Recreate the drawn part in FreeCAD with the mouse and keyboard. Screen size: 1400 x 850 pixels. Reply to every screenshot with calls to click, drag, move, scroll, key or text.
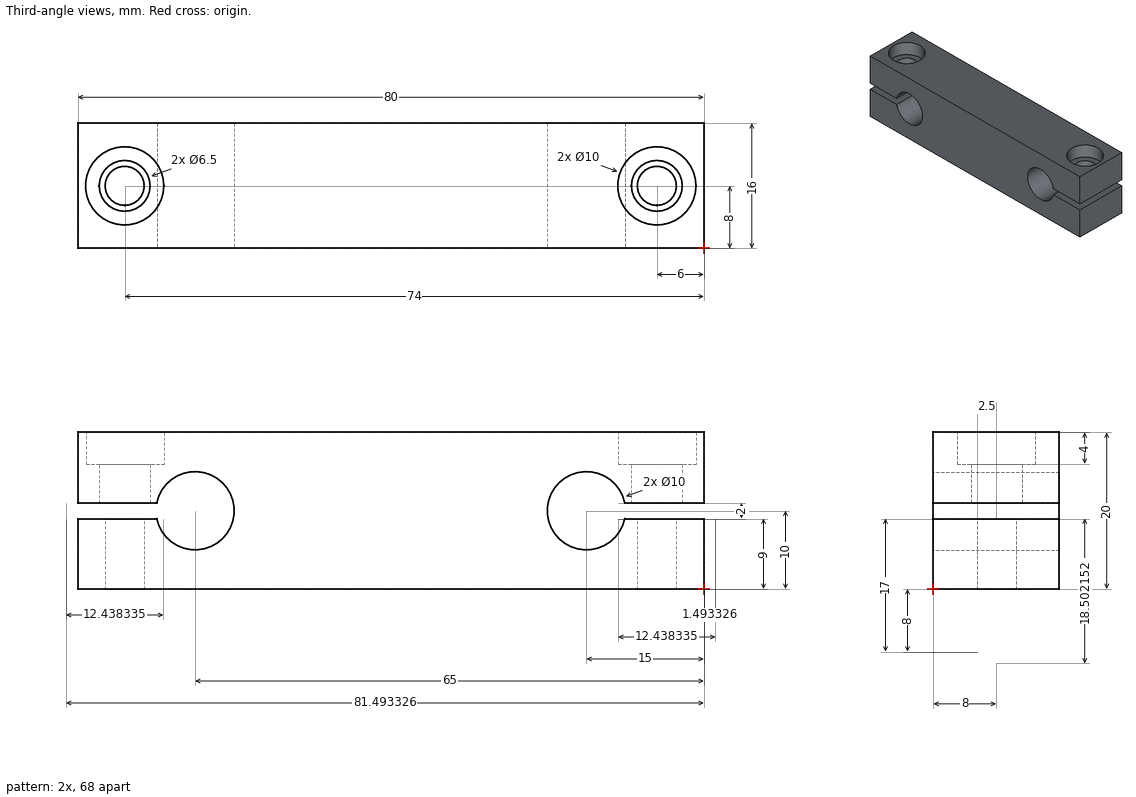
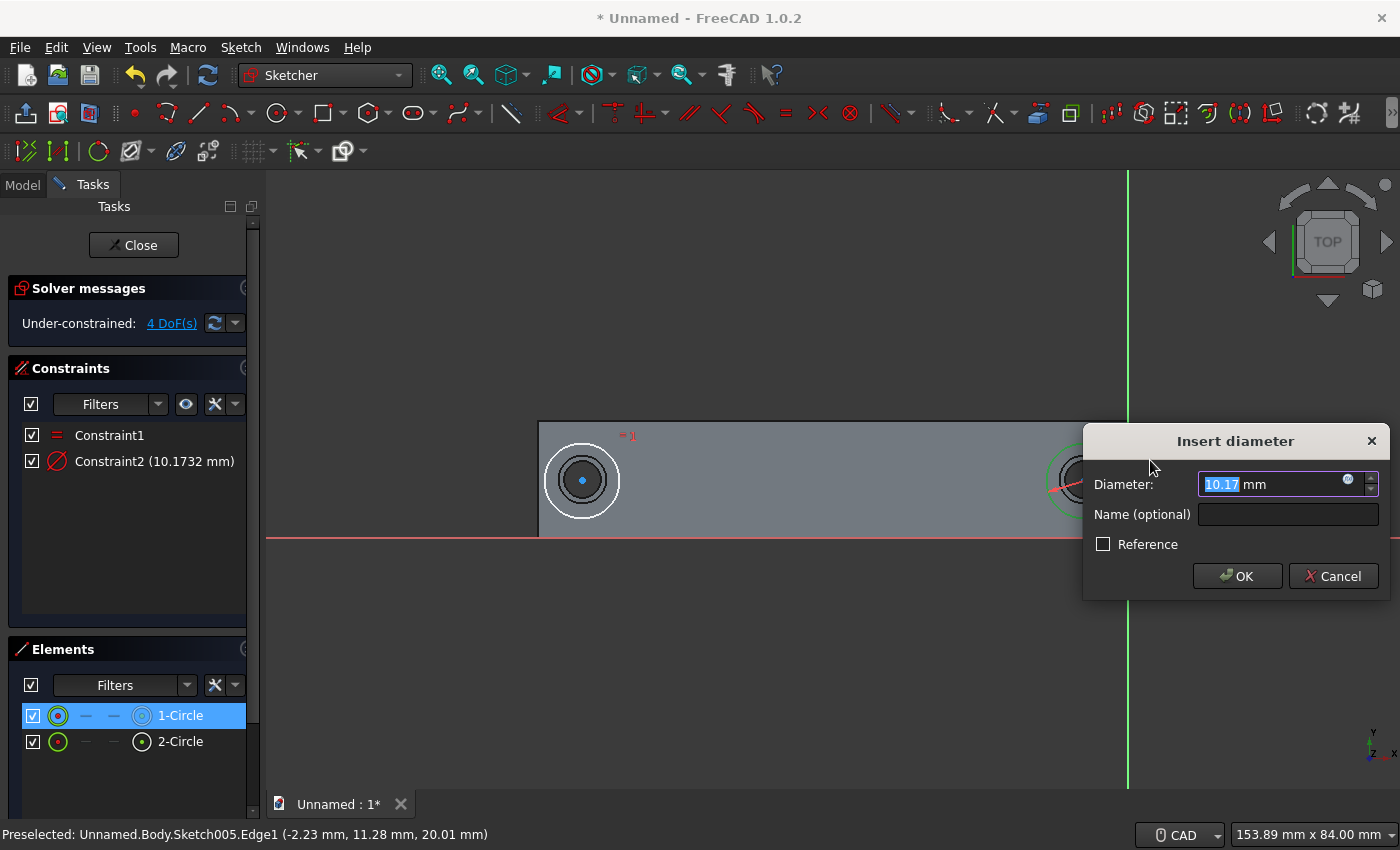
text(10)
key(Return)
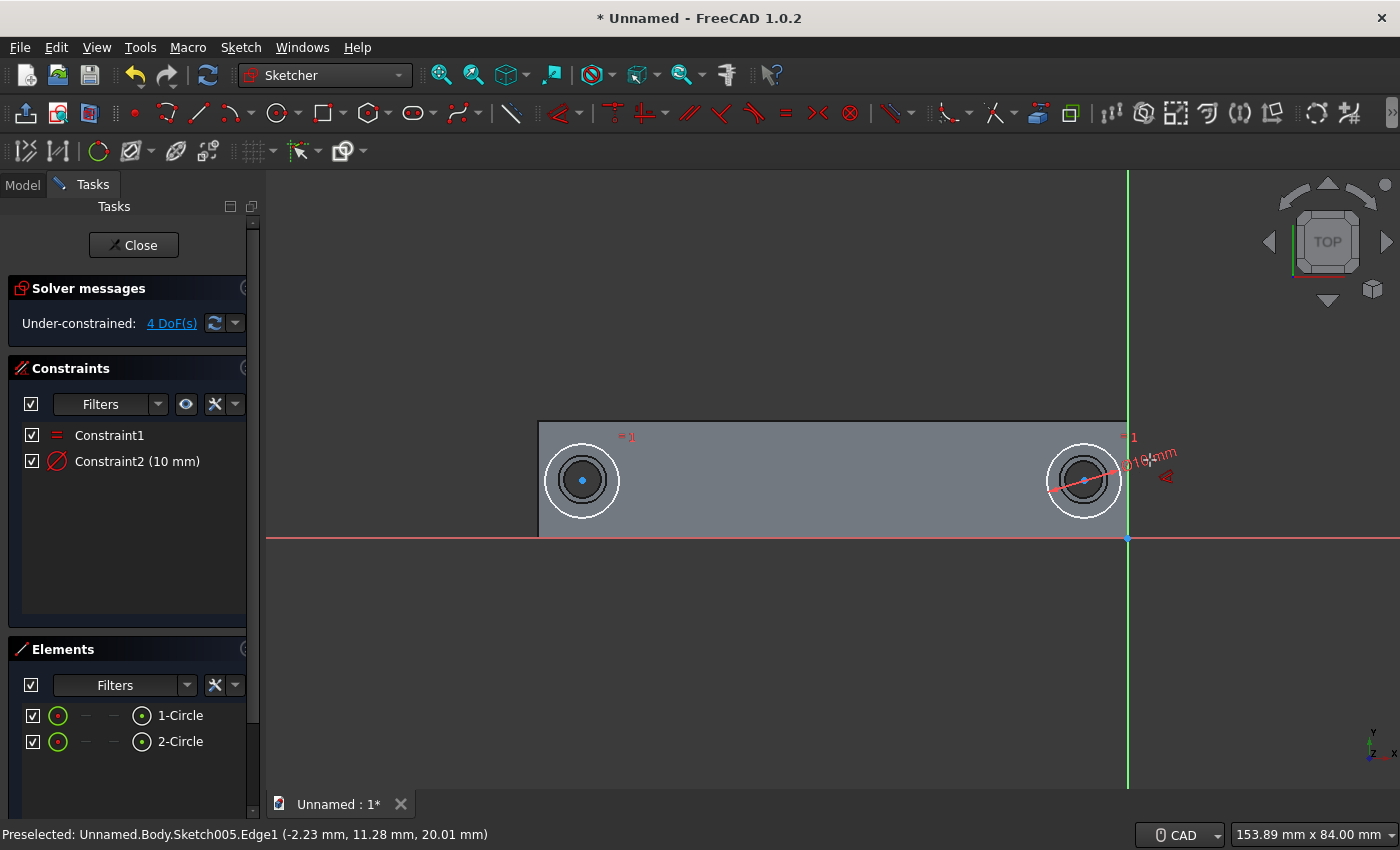
click(1084, 481)
click(1106, 572)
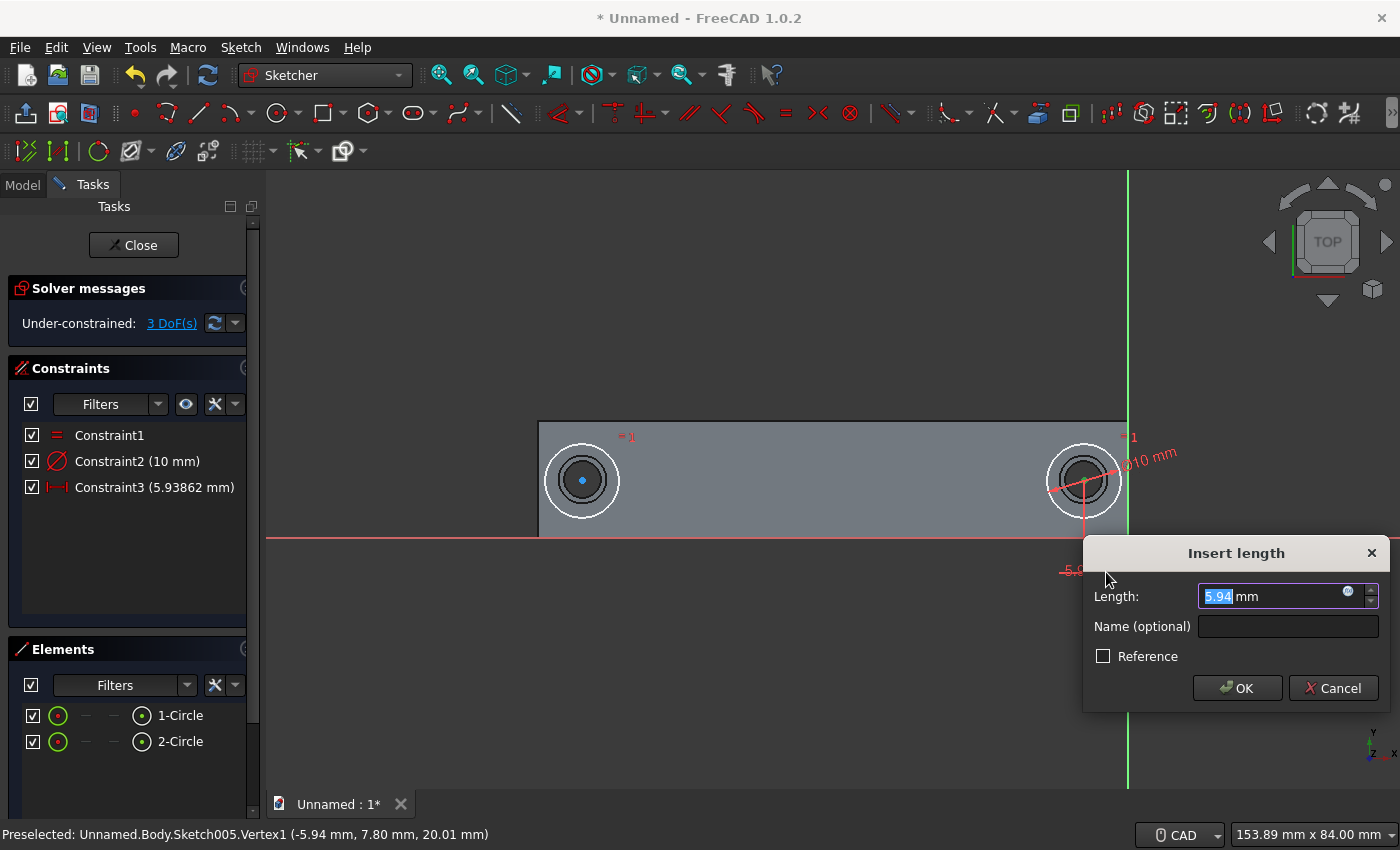
text(6)
key(Return)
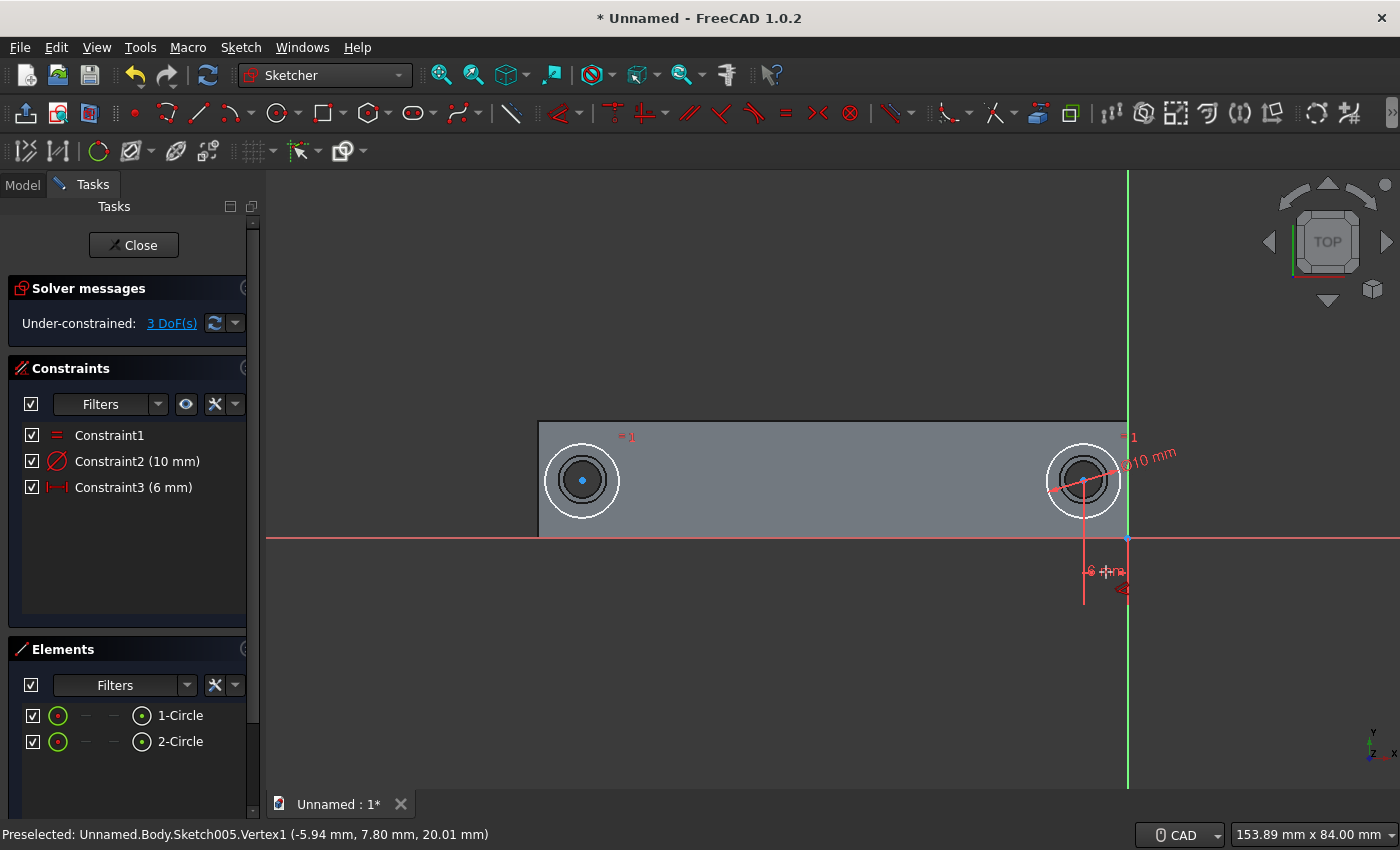
click(1084, 481)
click(1162, 510)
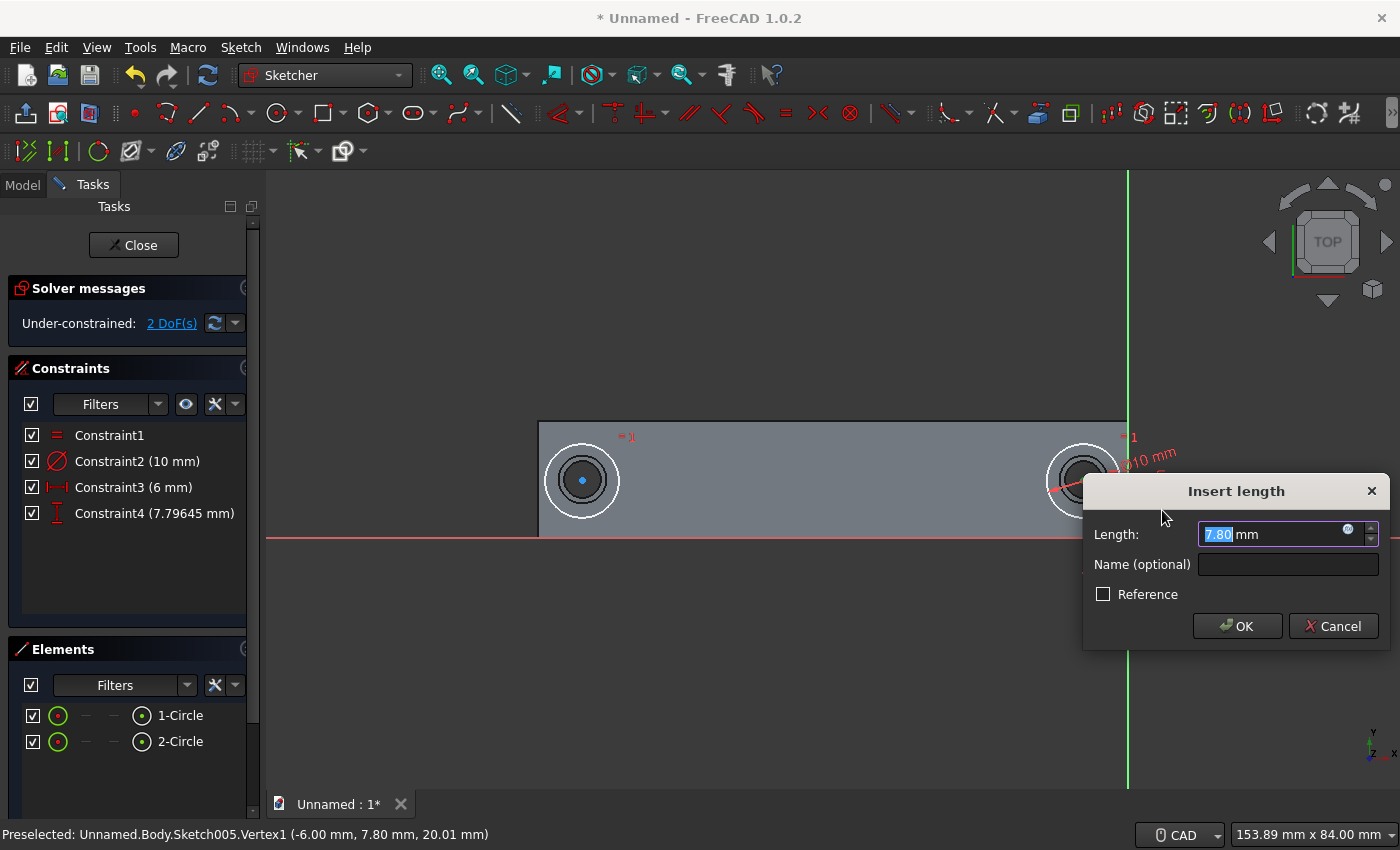
text(8)
key(Return)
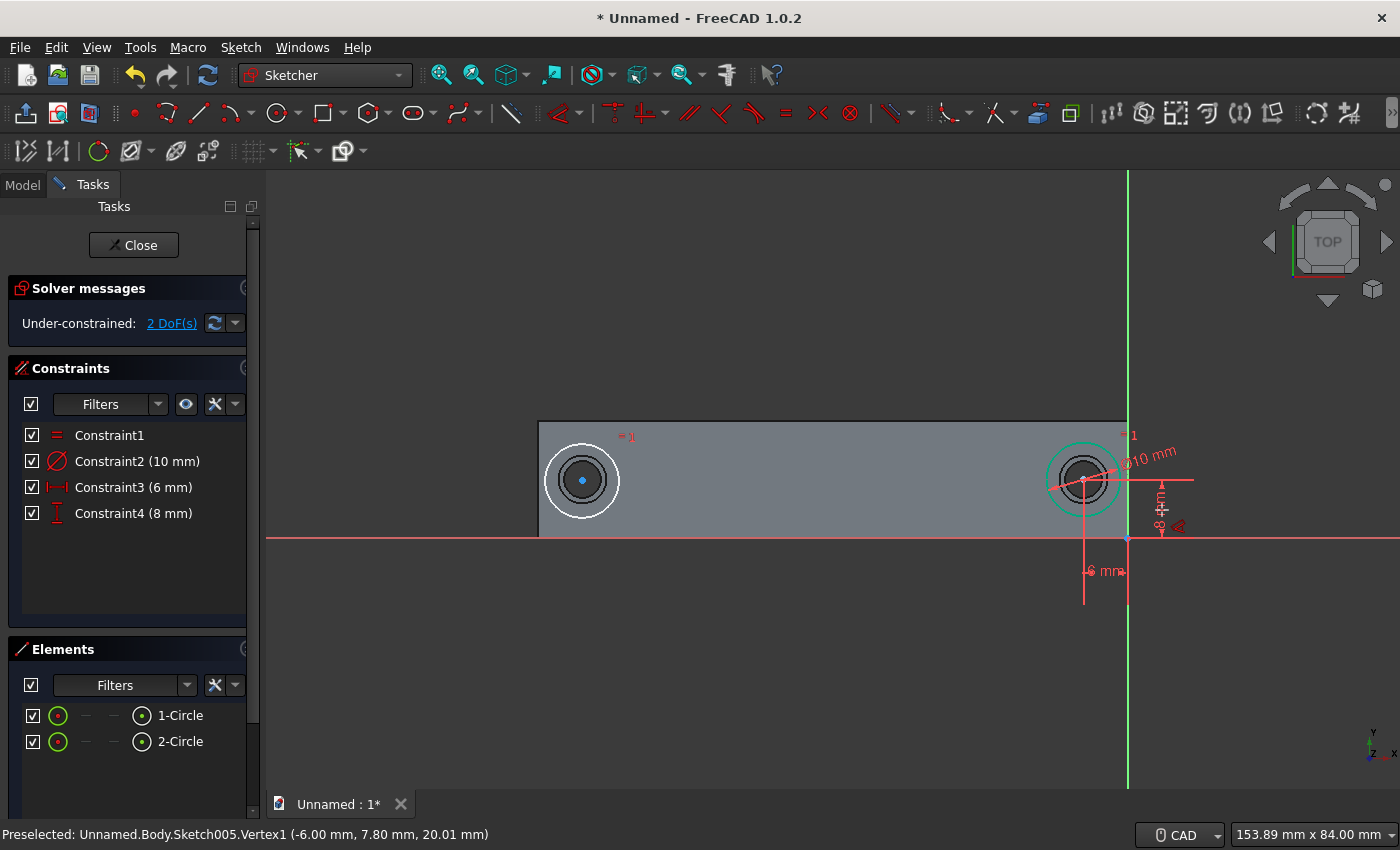
click(582, 481)
click(1162, 490)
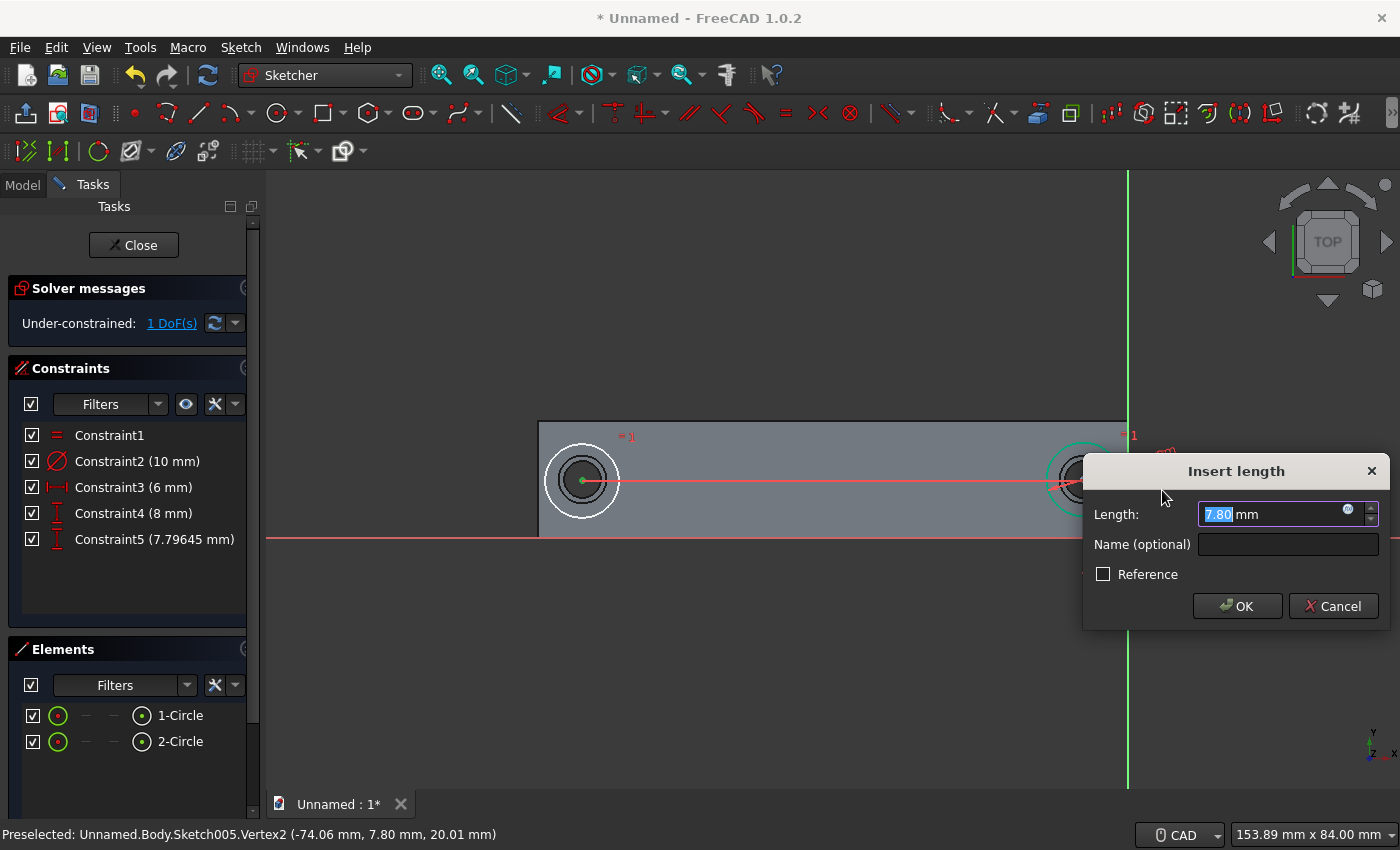
text(8)
key(Return)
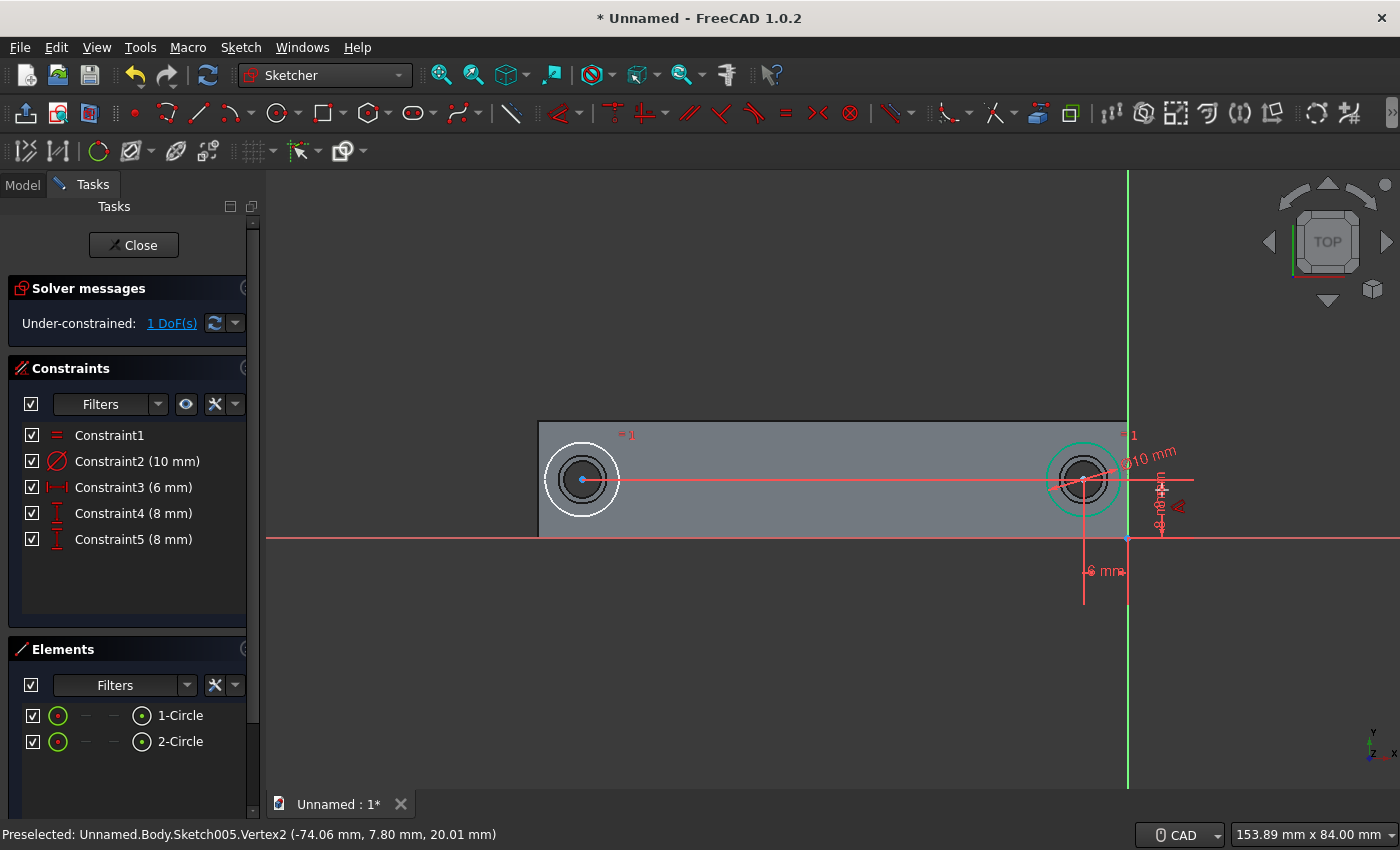
click(582, 480)
click(855, 572)